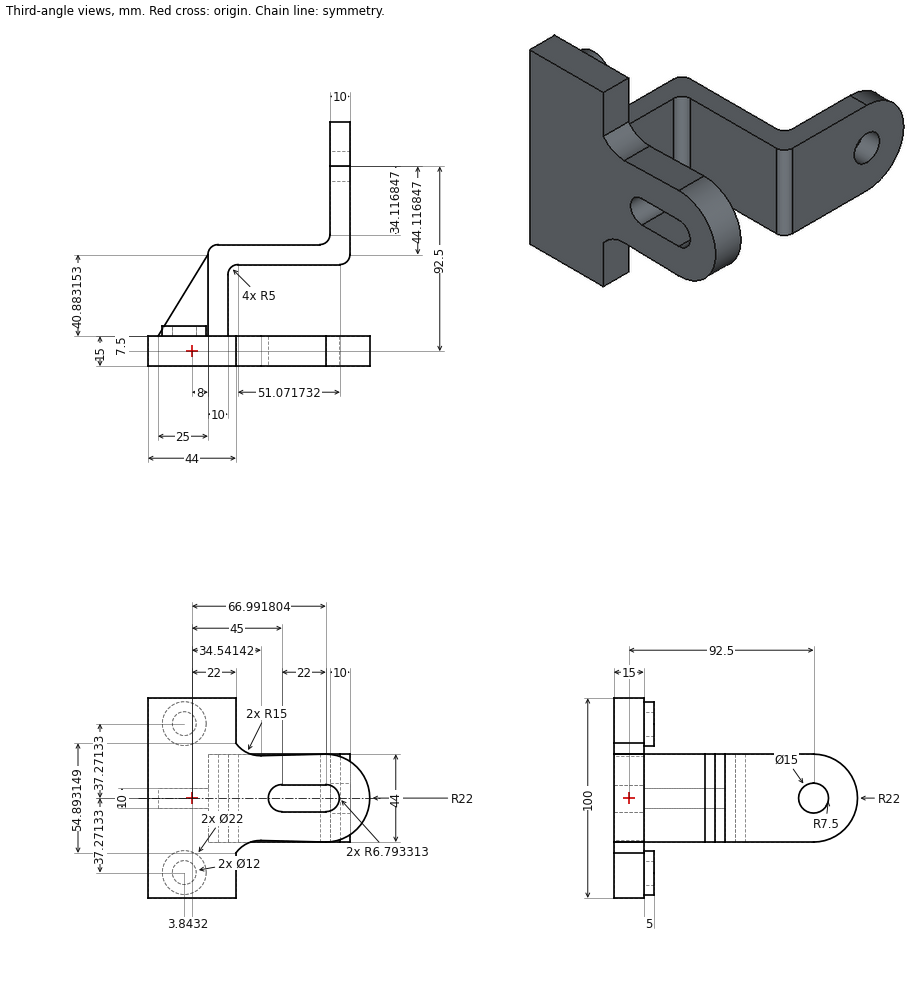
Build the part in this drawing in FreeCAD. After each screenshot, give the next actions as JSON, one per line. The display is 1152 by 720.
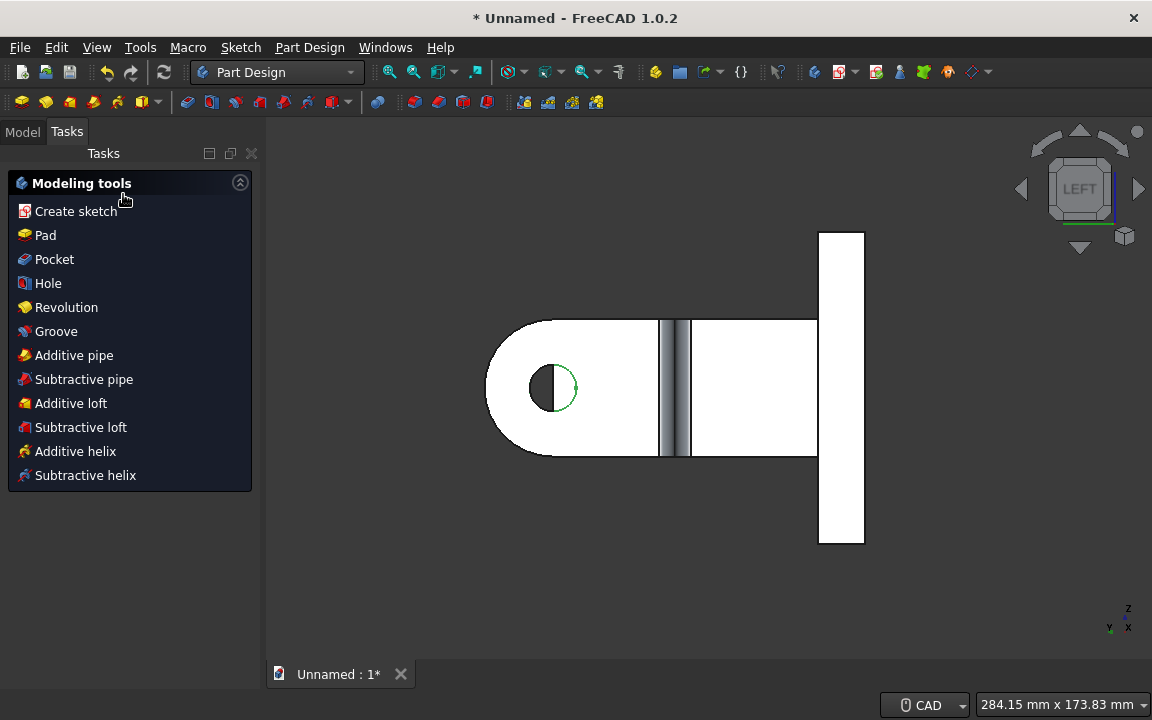
{"action": "left_click", "coordinate": [188, 102]}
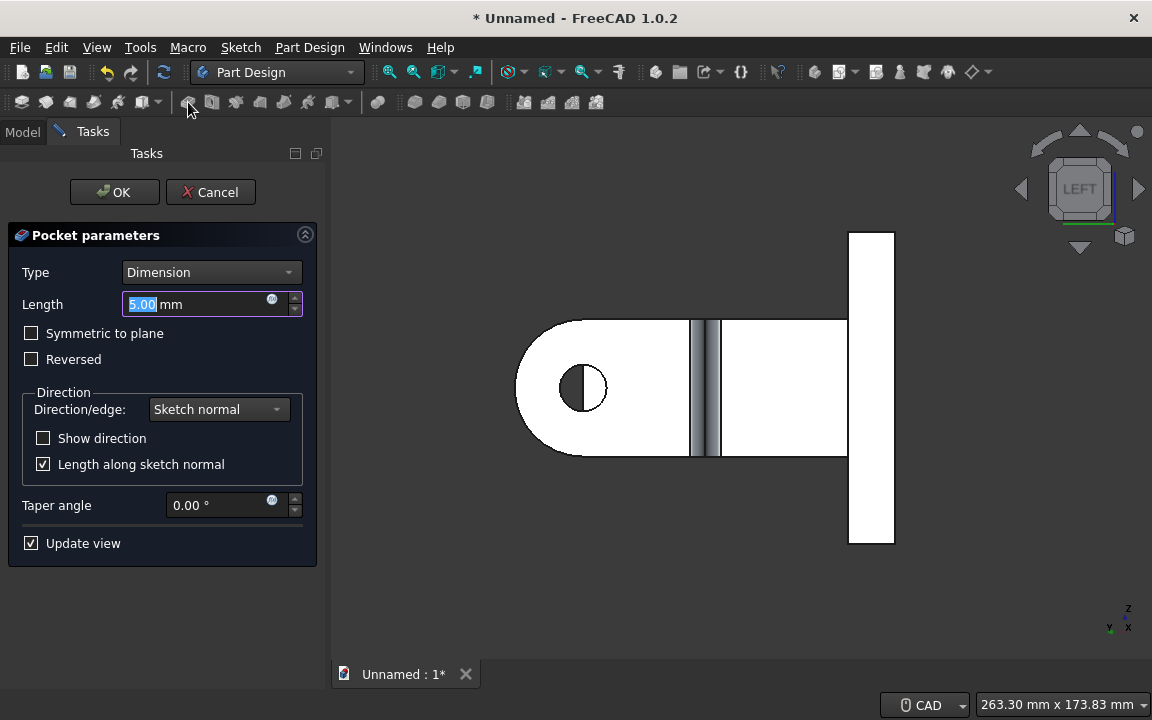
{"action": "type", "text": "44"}
{"action": "key", "text": "Tab"}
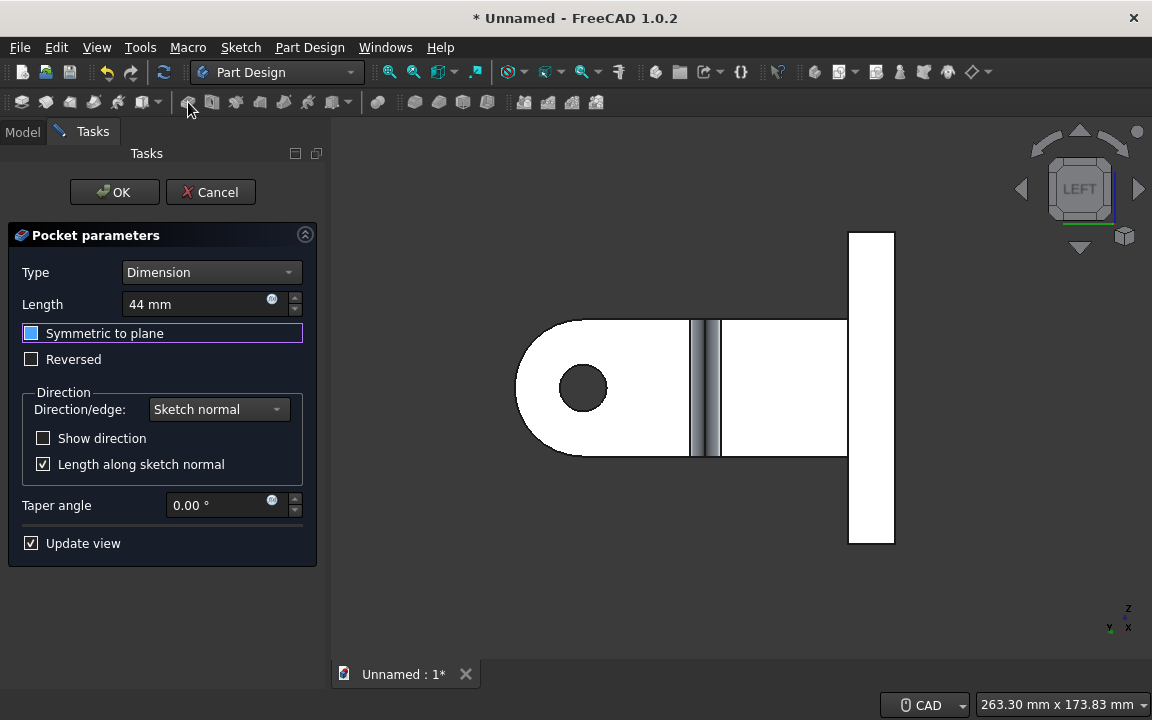
{"action": "left_click", "coordinate": [115, 192]}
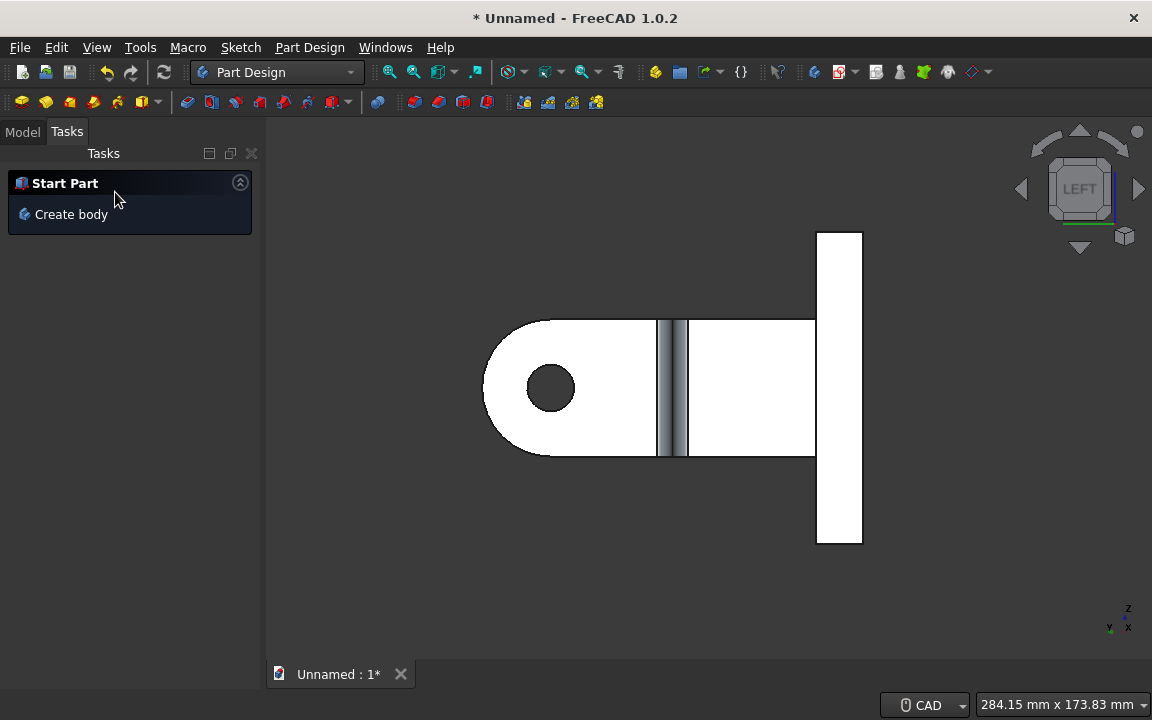
{"action": "key", "text": "4"}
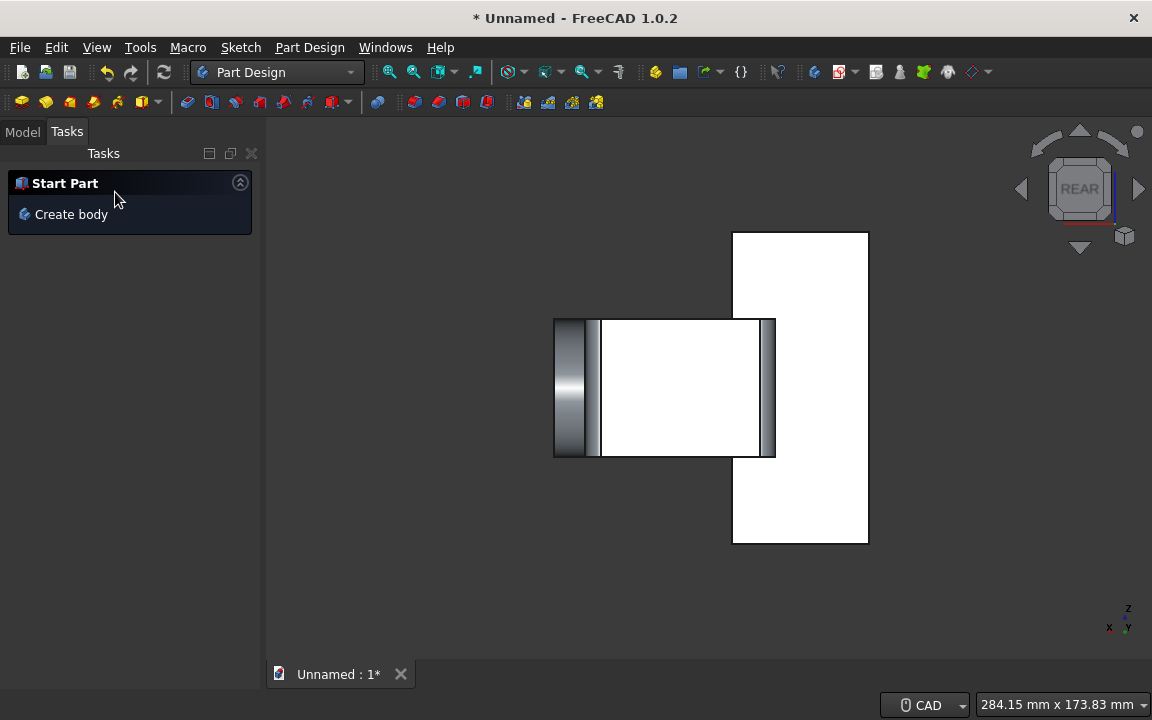
{"action": "left_click", "coordinate": [820, 298]}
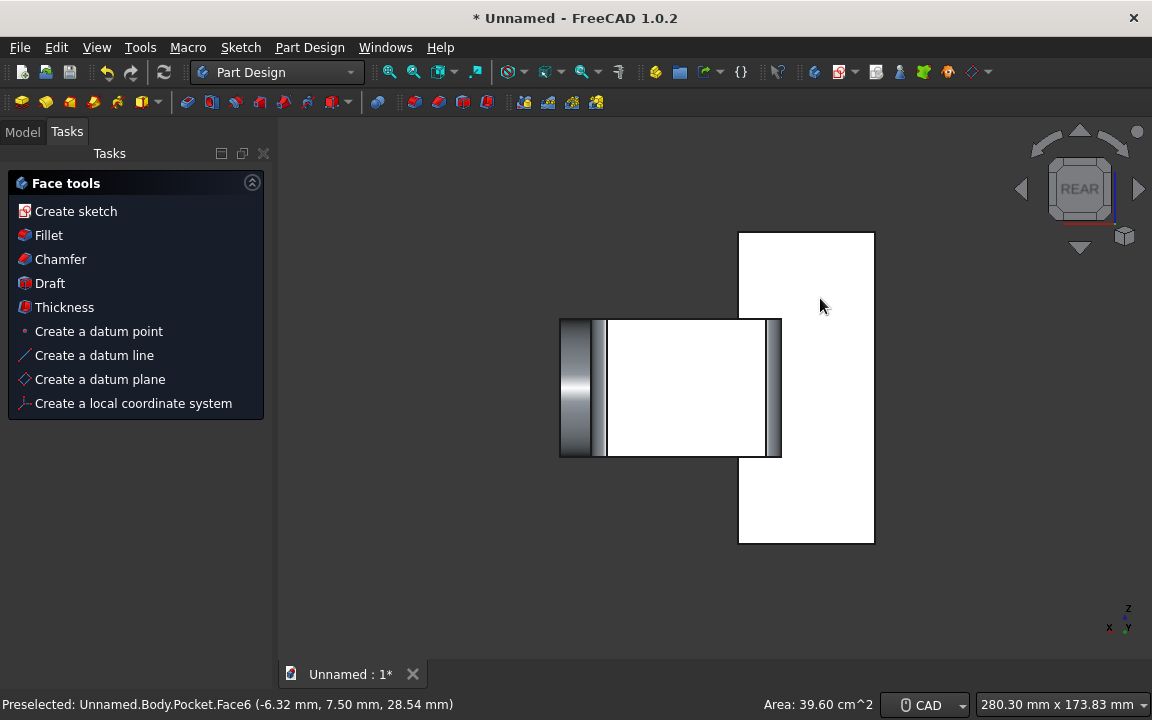
{"action": "left_click", "coordinate": [840, 72]}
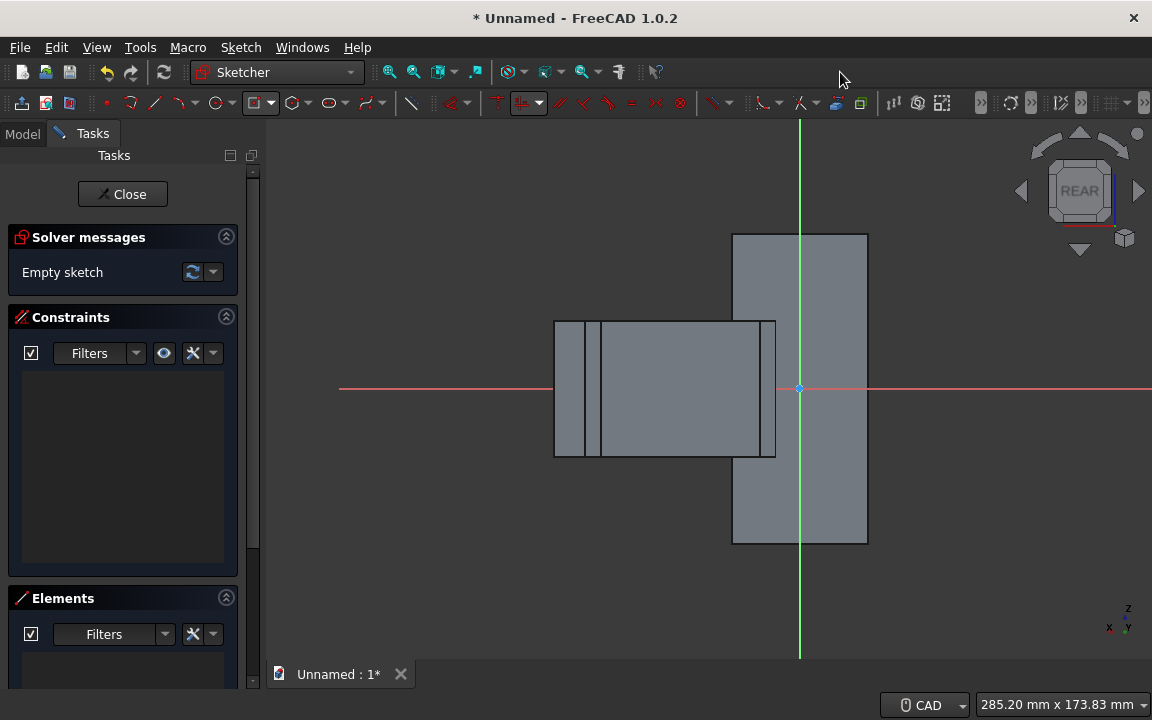
{"action": "left_click", "coordinate": [70, 104]}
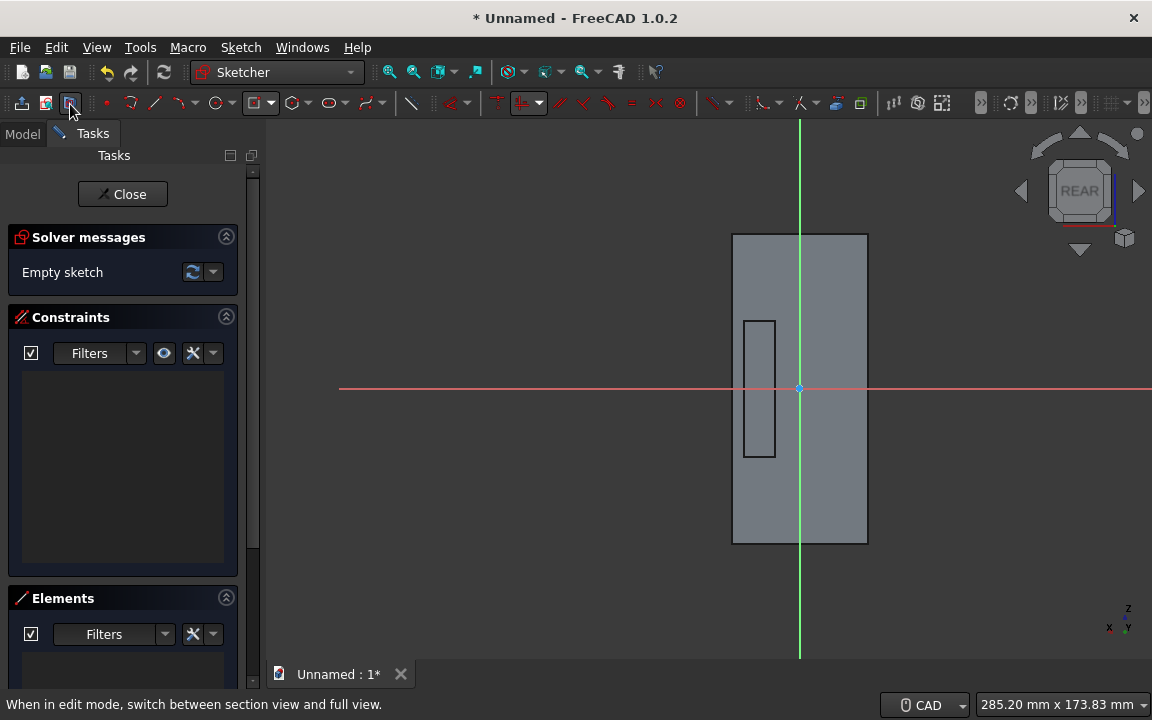
{"action": "left_click", "coordinate": [216, 104]}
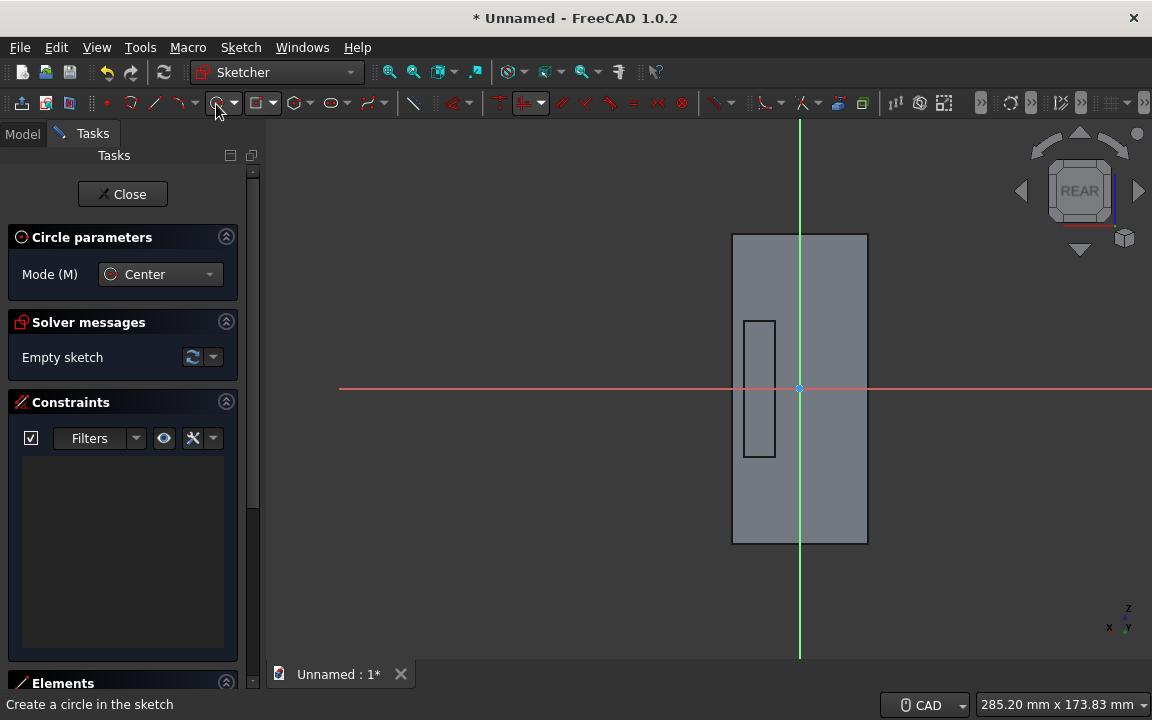
{"action": "scroll", "coordinate": [812, 505], "scroll_direction": "up", "scroll_amount": 2}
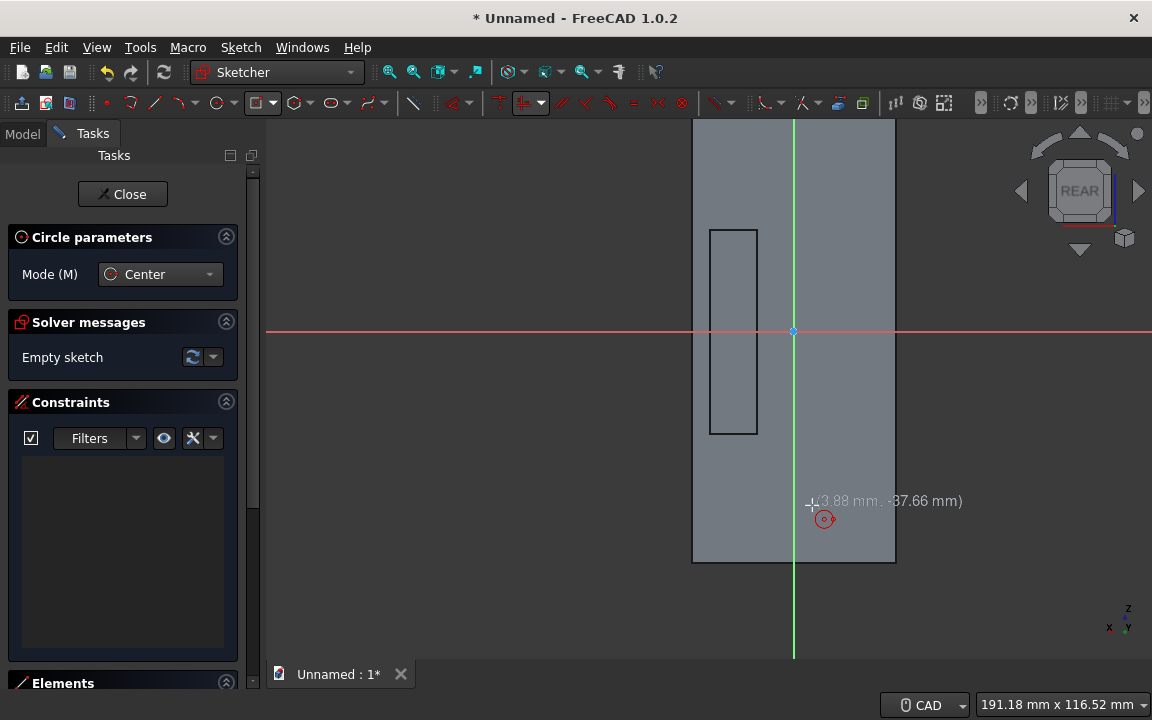
{"action": "left_click", "coordinate": [812, 504]}
{"action": "mouse_move", "coordinate": [848, 468]}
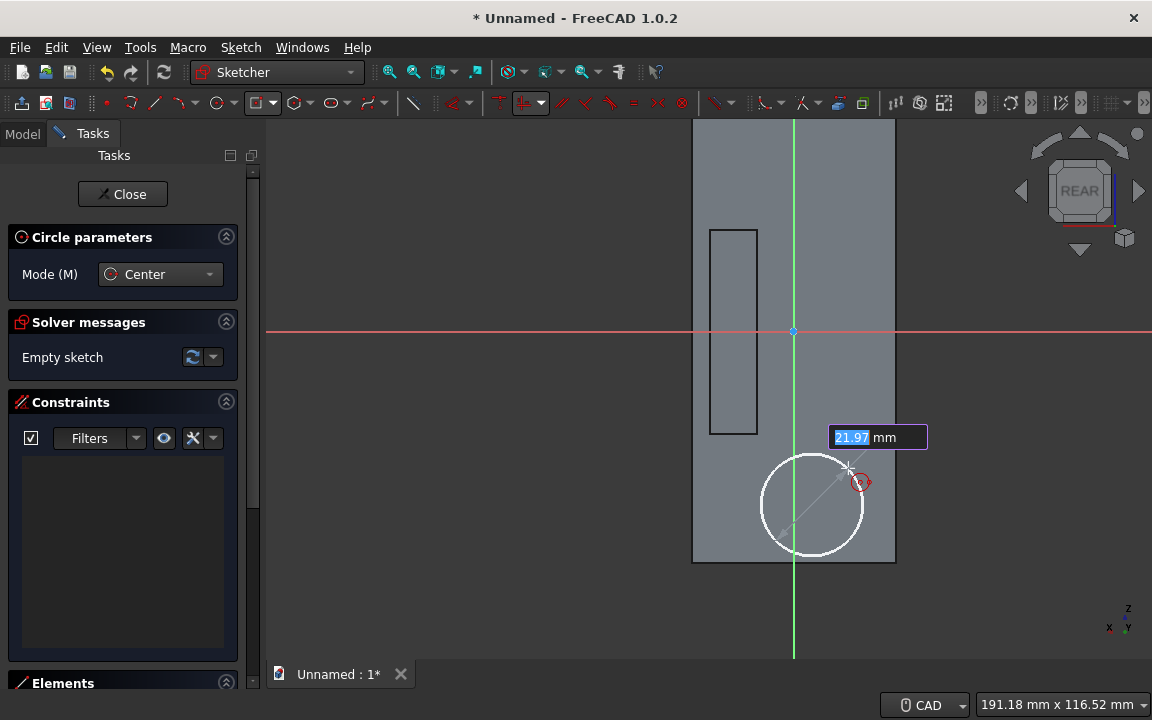
{"action": "type", "text": "22"}
{"action": "key", "text": "Return"}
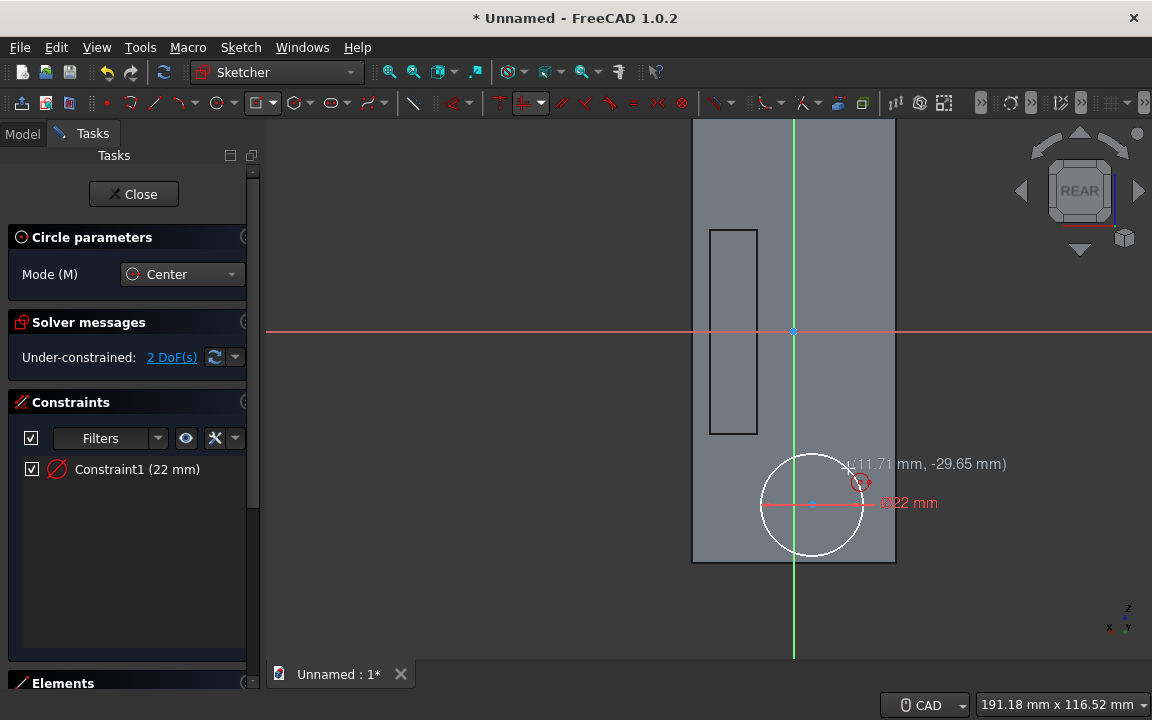
{"action": "left_click", "coordinate": [812, 159]}